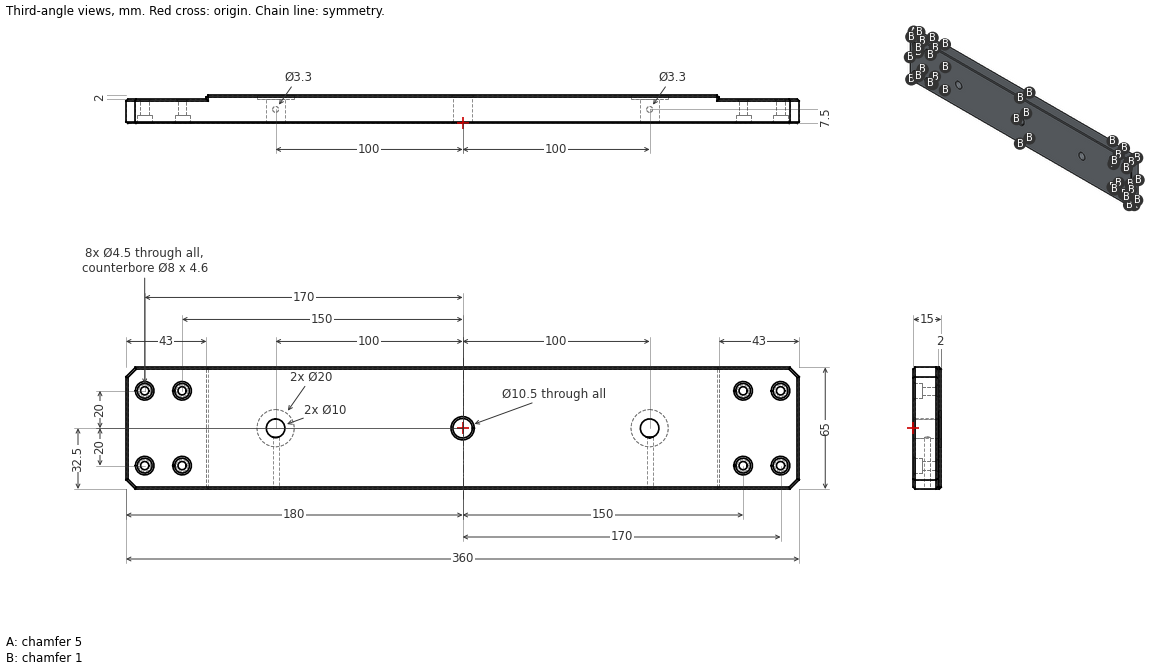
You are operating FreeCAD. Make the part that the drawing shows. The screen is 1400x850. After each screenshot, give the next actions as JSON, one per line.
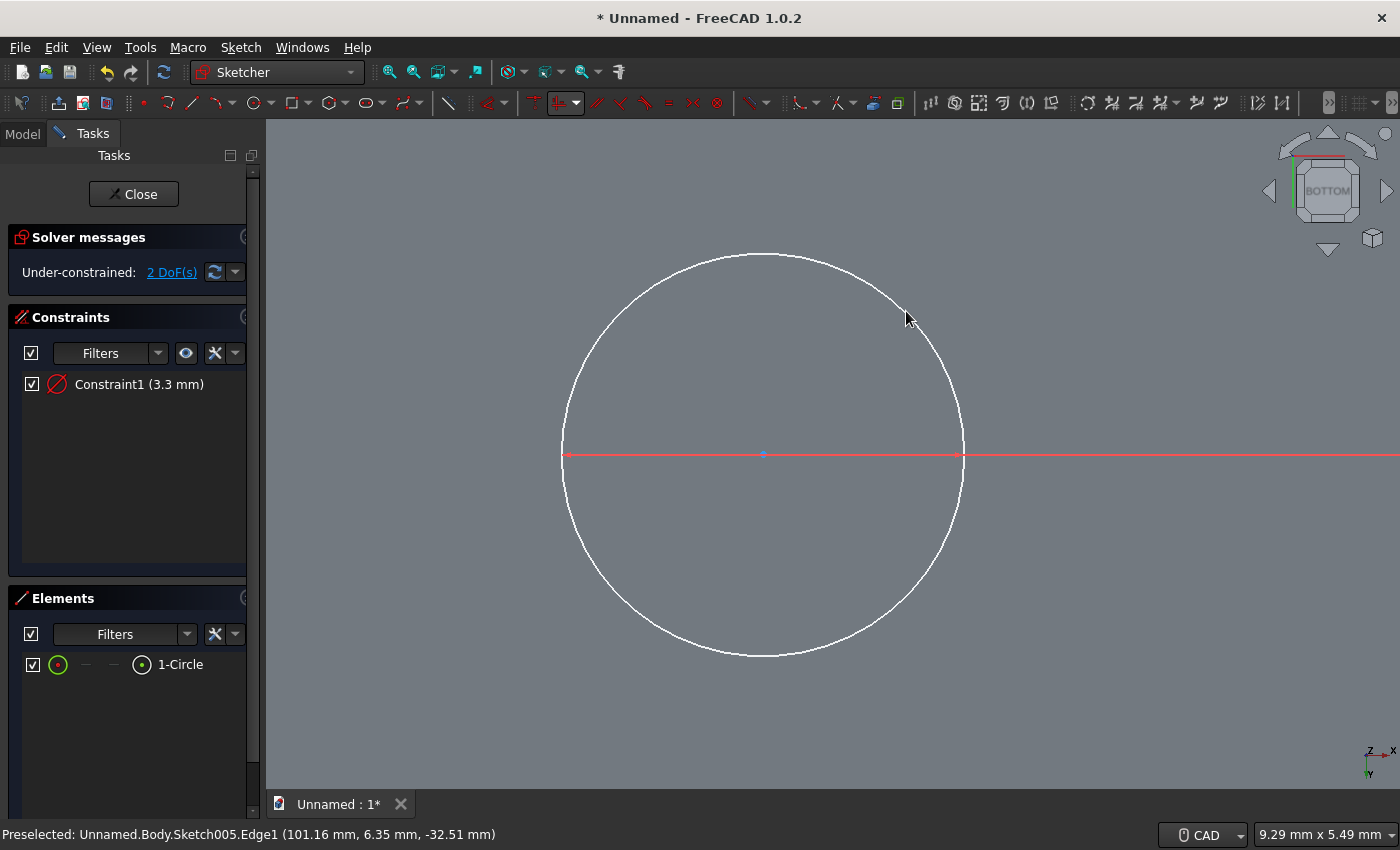
{"action": "key", "text": "d"}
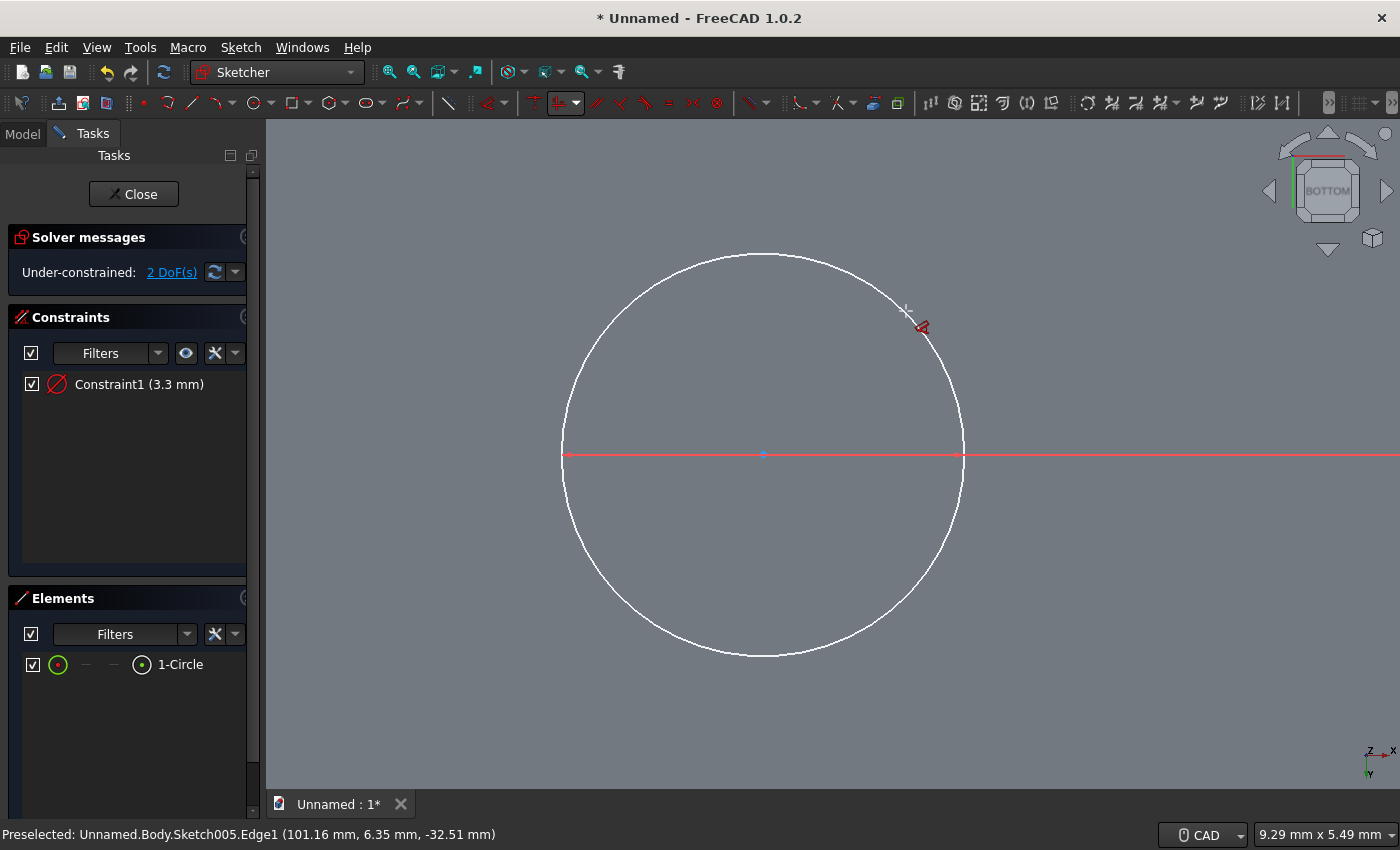
{"action": "left_click", "coordinate": [763, 455]}
{"action": "left_click", "coordinate": [528, 489]}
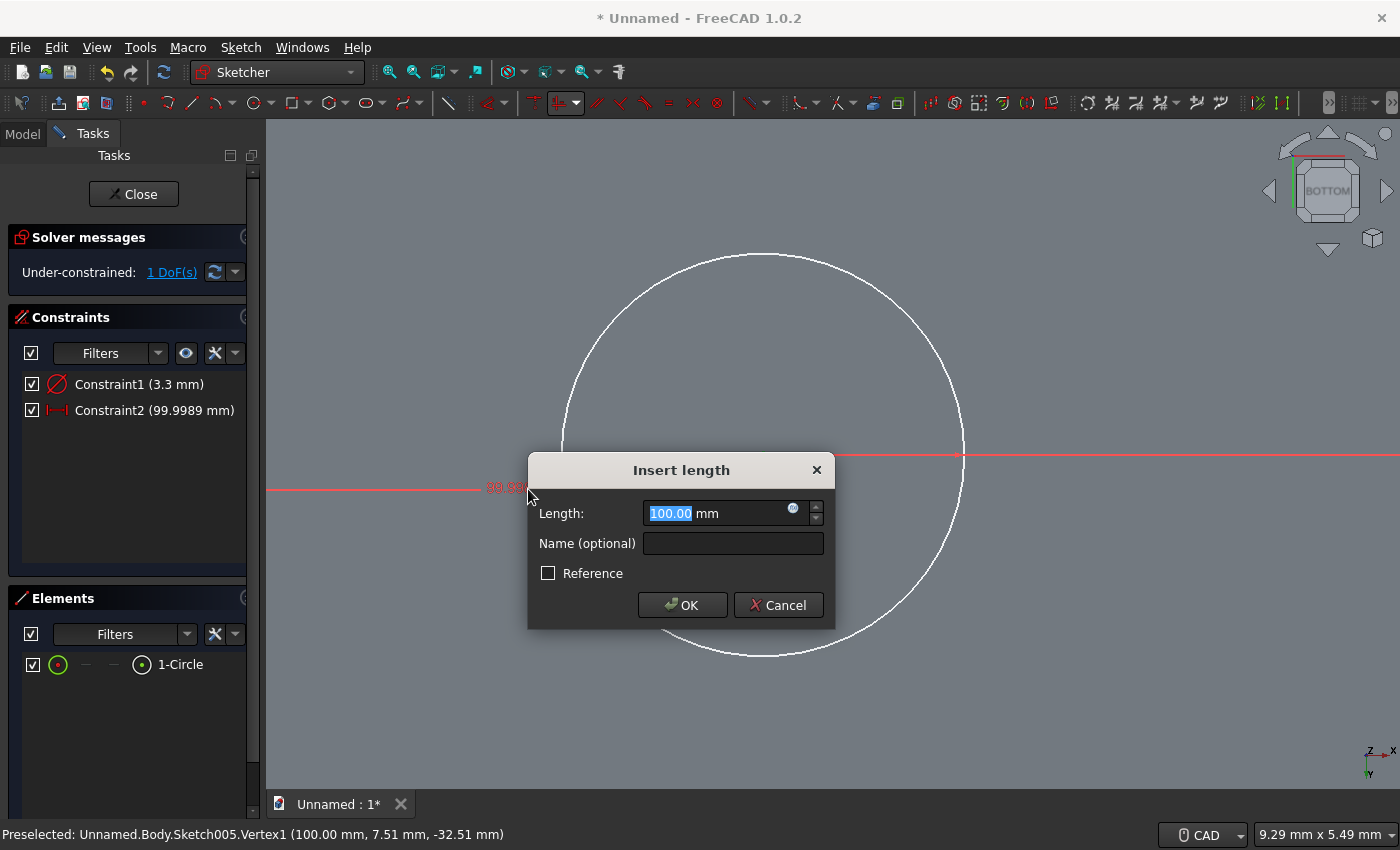
{"action": "type", "text": "100"}
{"action": "key", "text": "Return"}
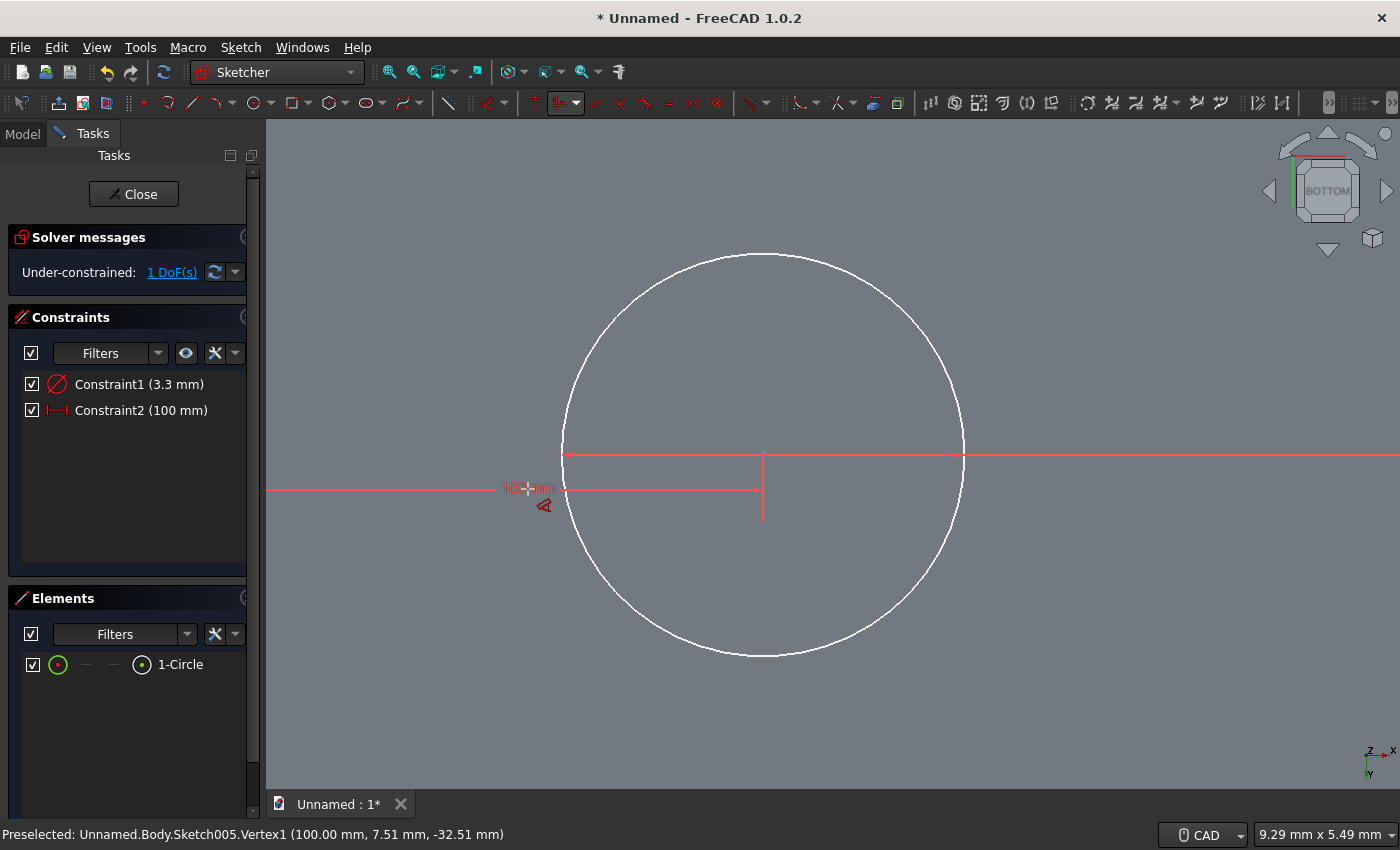
{"action": "left_click", "coordinate": [763, 455]}
{"action": "left_click", "coordinate": [797, 301]}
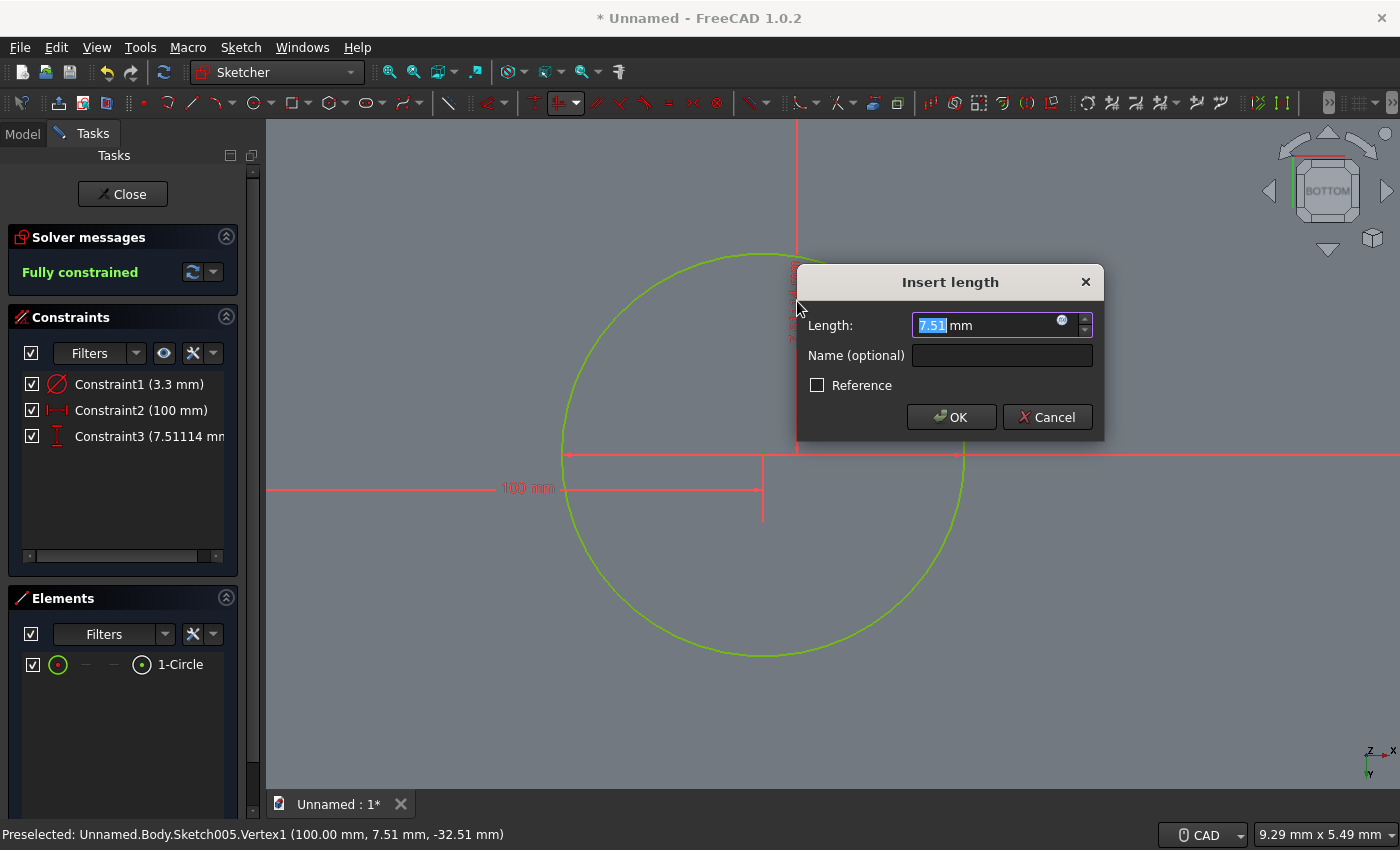
{"action": "type", "text": "7.5"}
{"action": "key", "text": "Return"}
{"action": "key", "text": "Escape"}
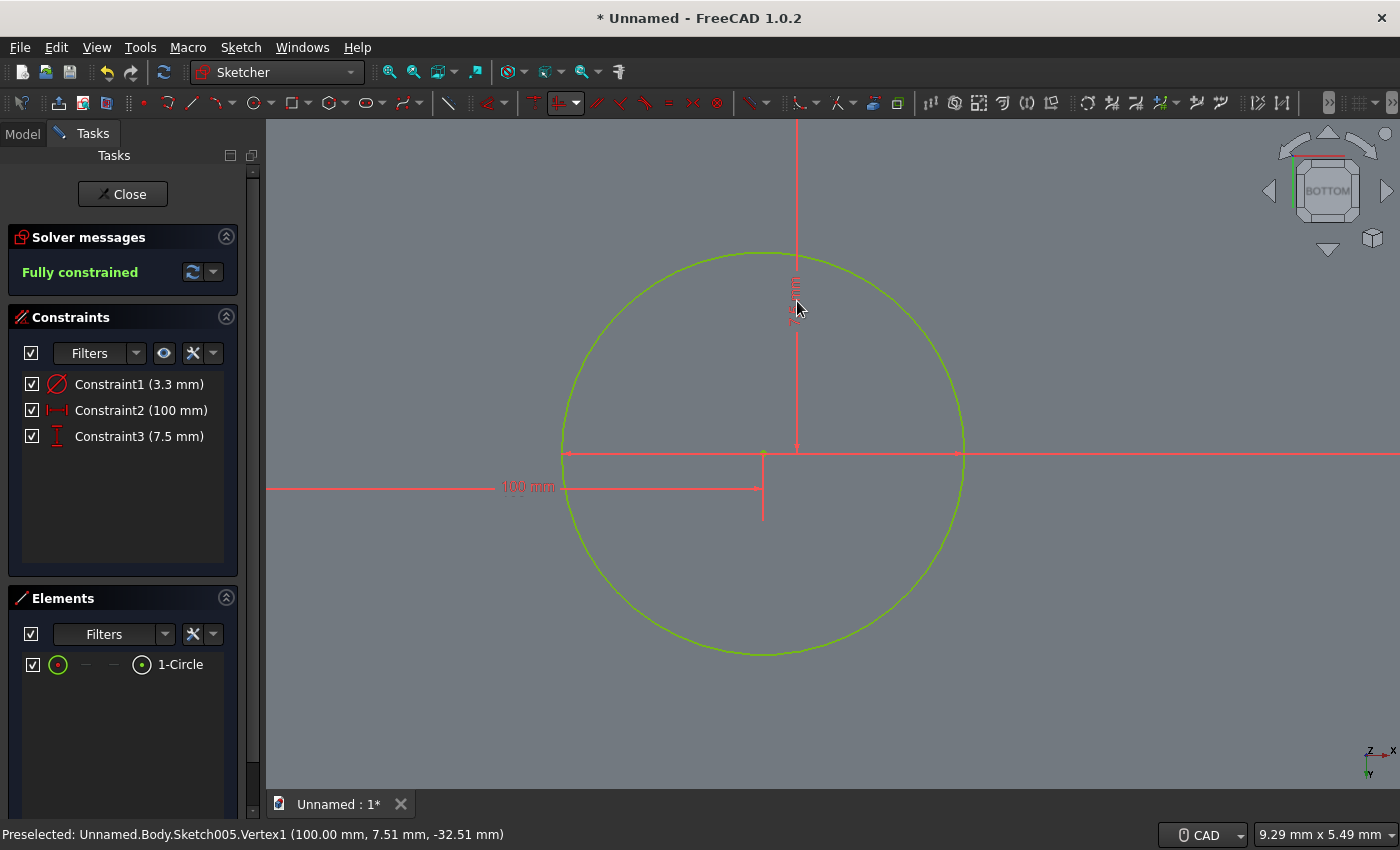
{"action": "left_click", "coordinate": [123, 194]}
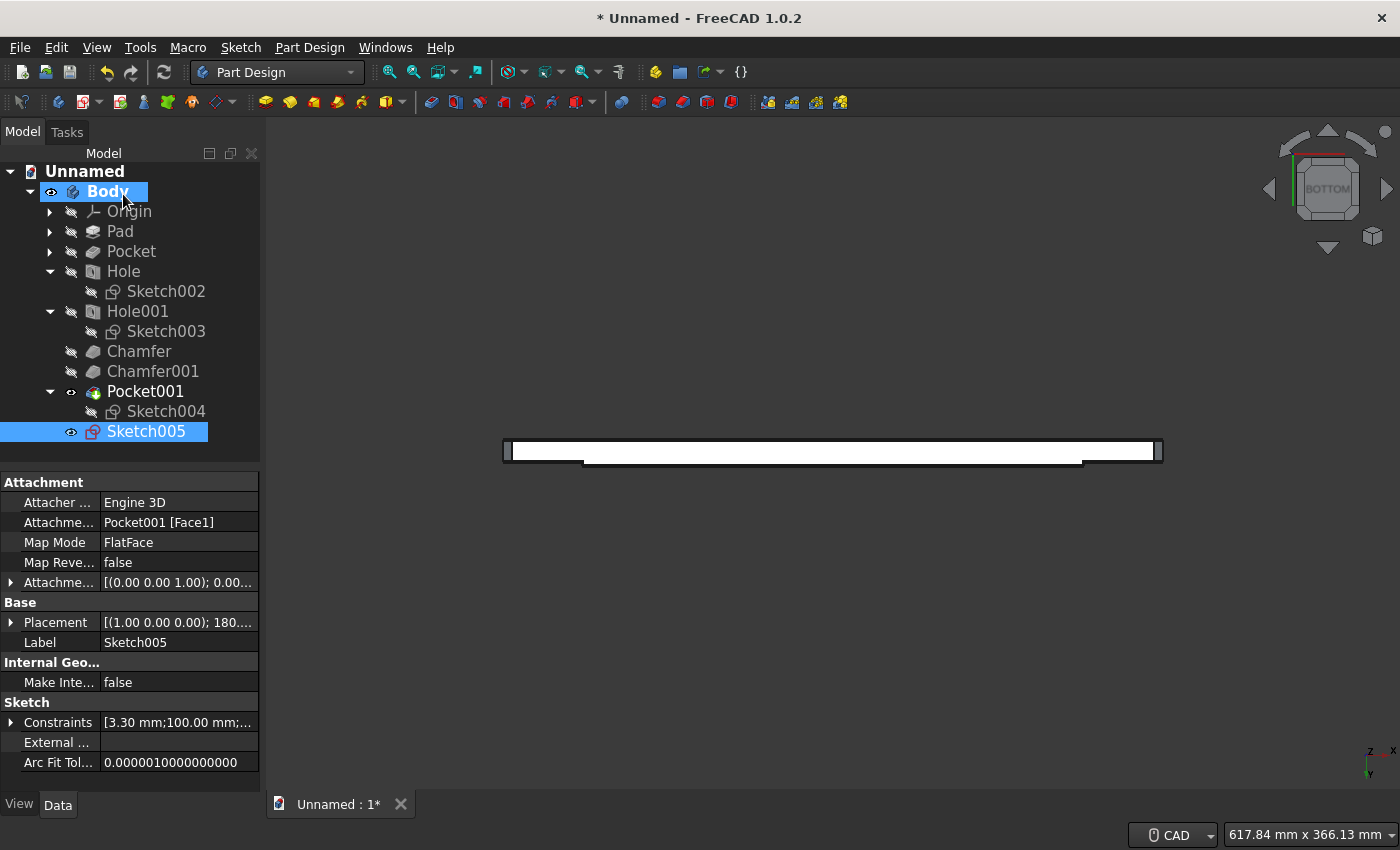
{"action": "left_click", "coordinate": [432, 102]}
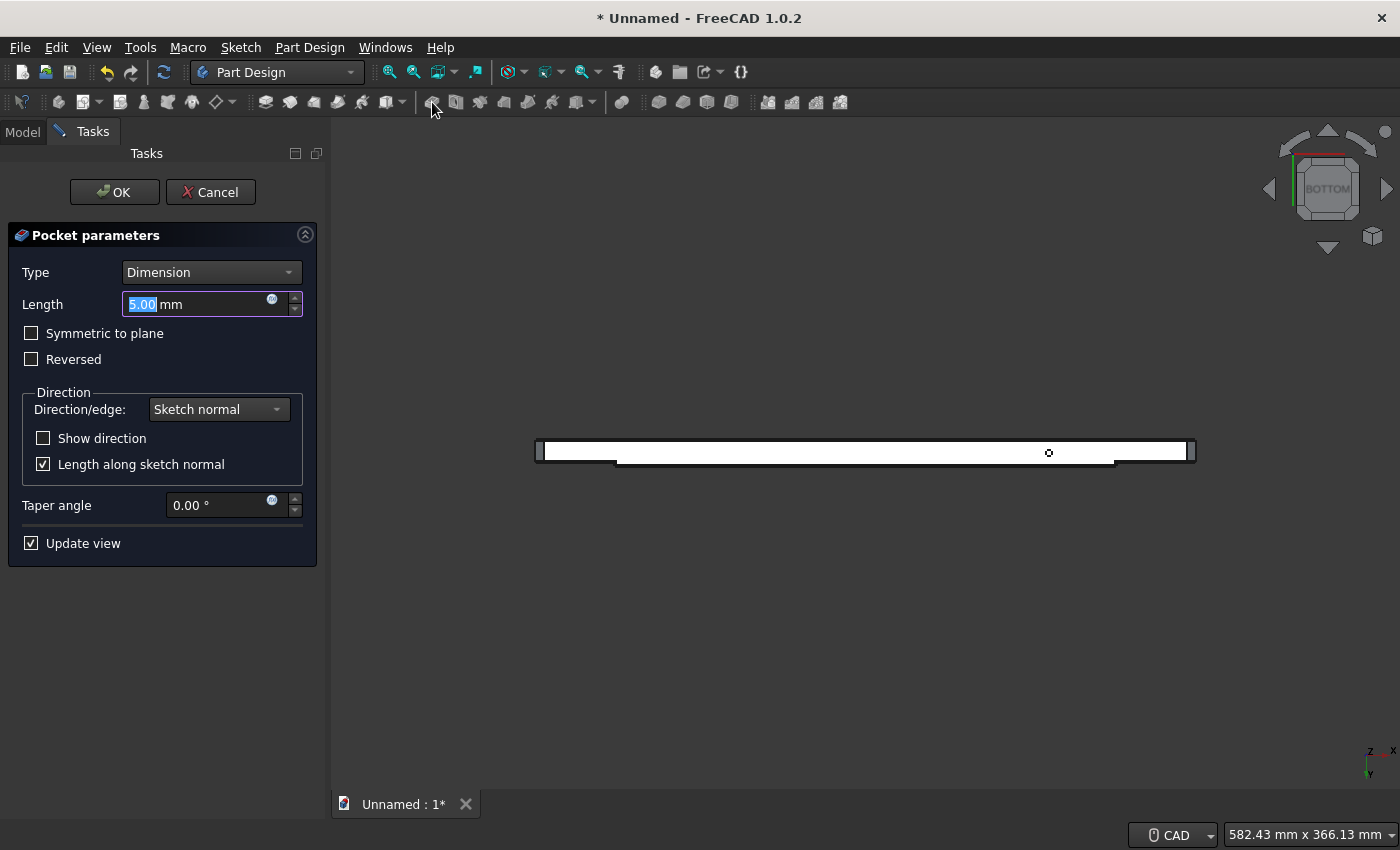
{"action": "left_click", "coordinate": [212, 272]}